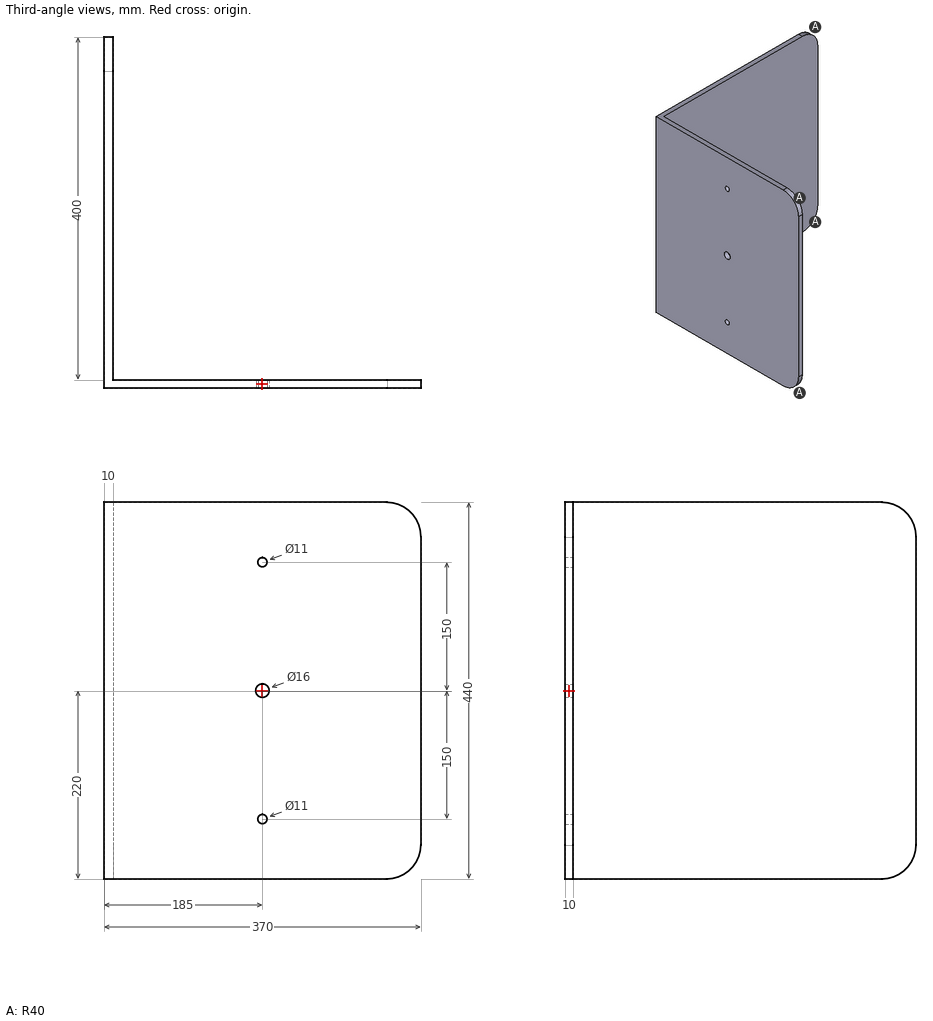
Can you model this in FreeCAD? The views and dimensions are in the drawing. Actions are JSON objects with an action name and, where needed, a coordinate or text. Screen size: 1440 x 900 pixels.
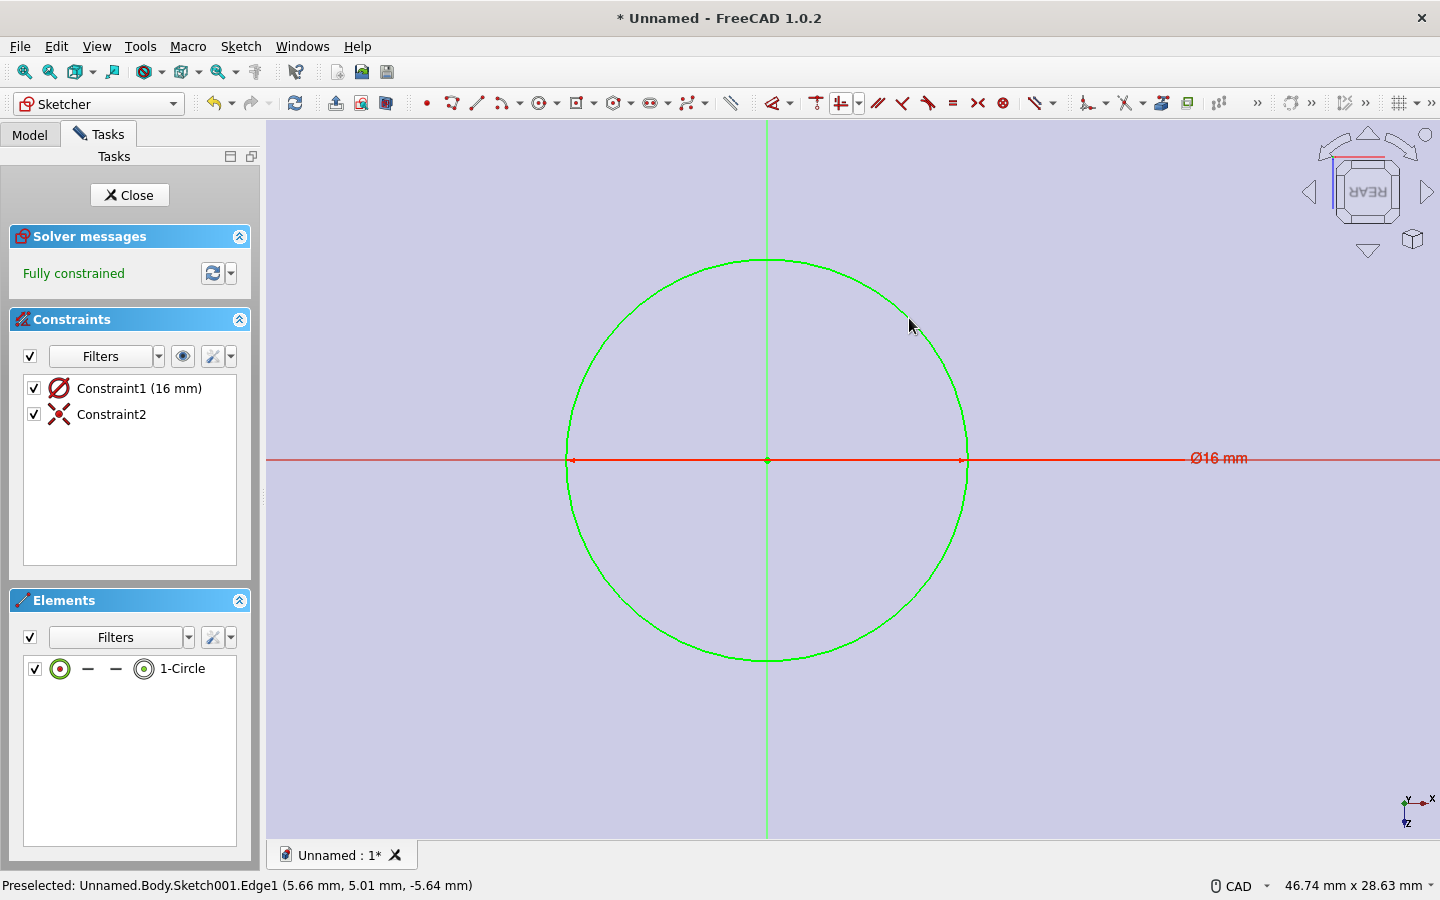
{"action": "left_click", "coordinate": [130, 195]}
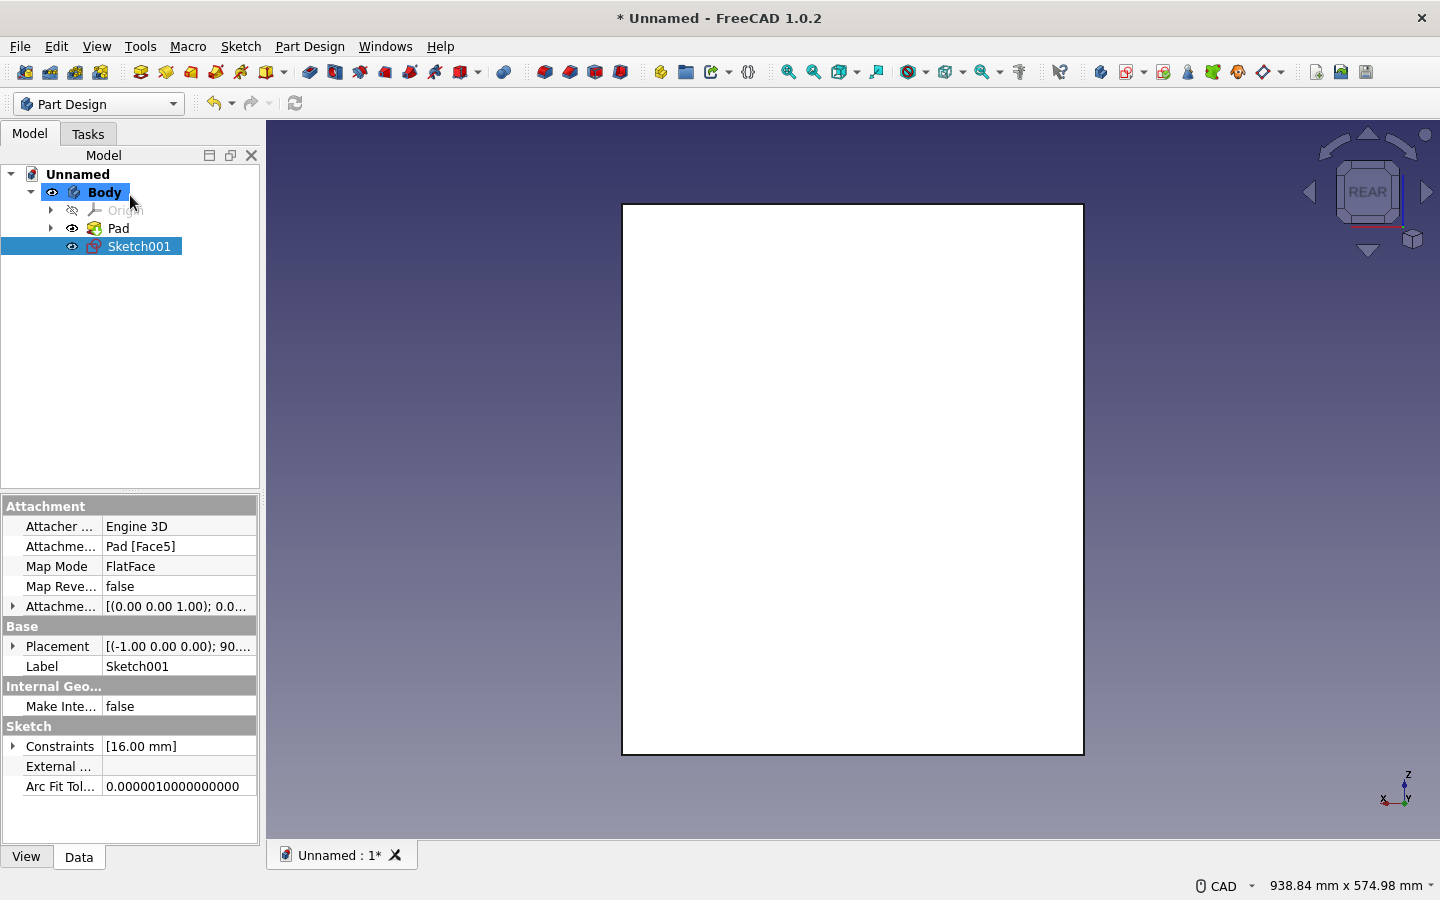
{"action": "left_click", "coordinate": [310, 72]}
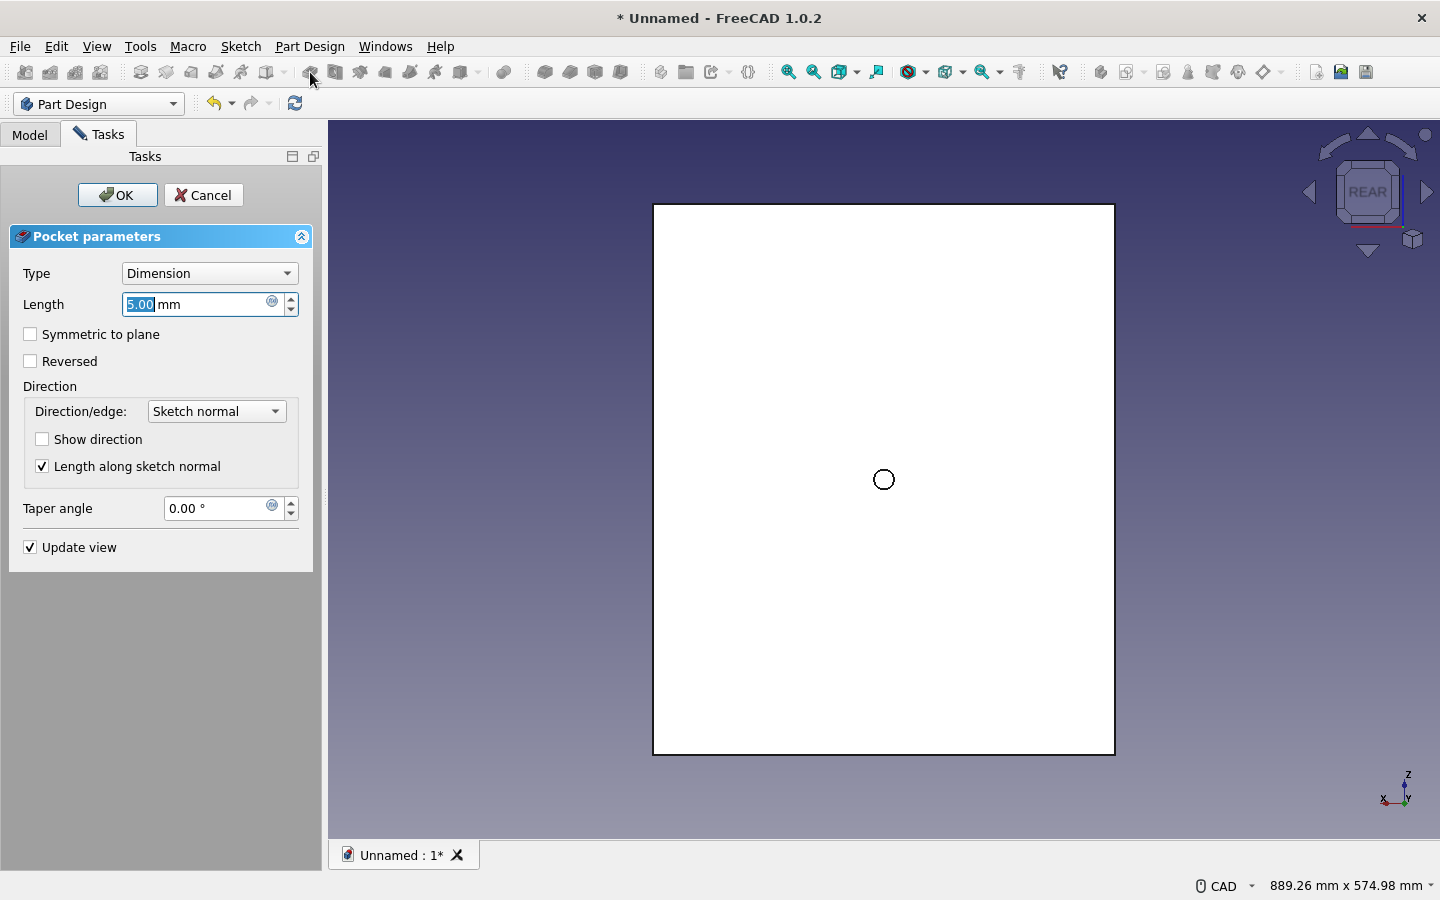
{"action": "left_click", "coordinate": [210, 274]}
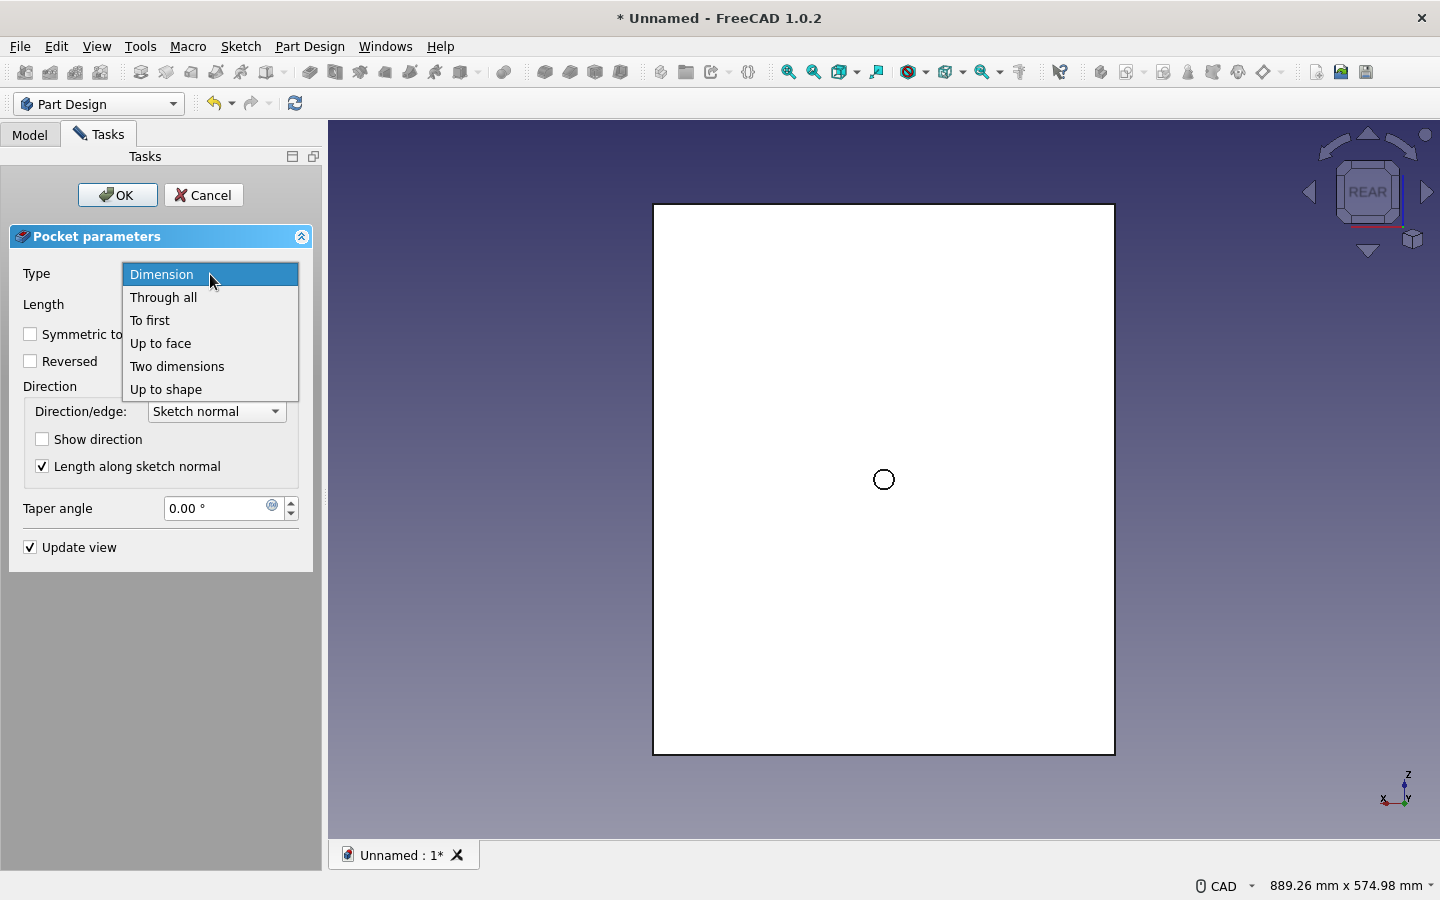
{"action": "left_click", "coordinate": [208, 320]}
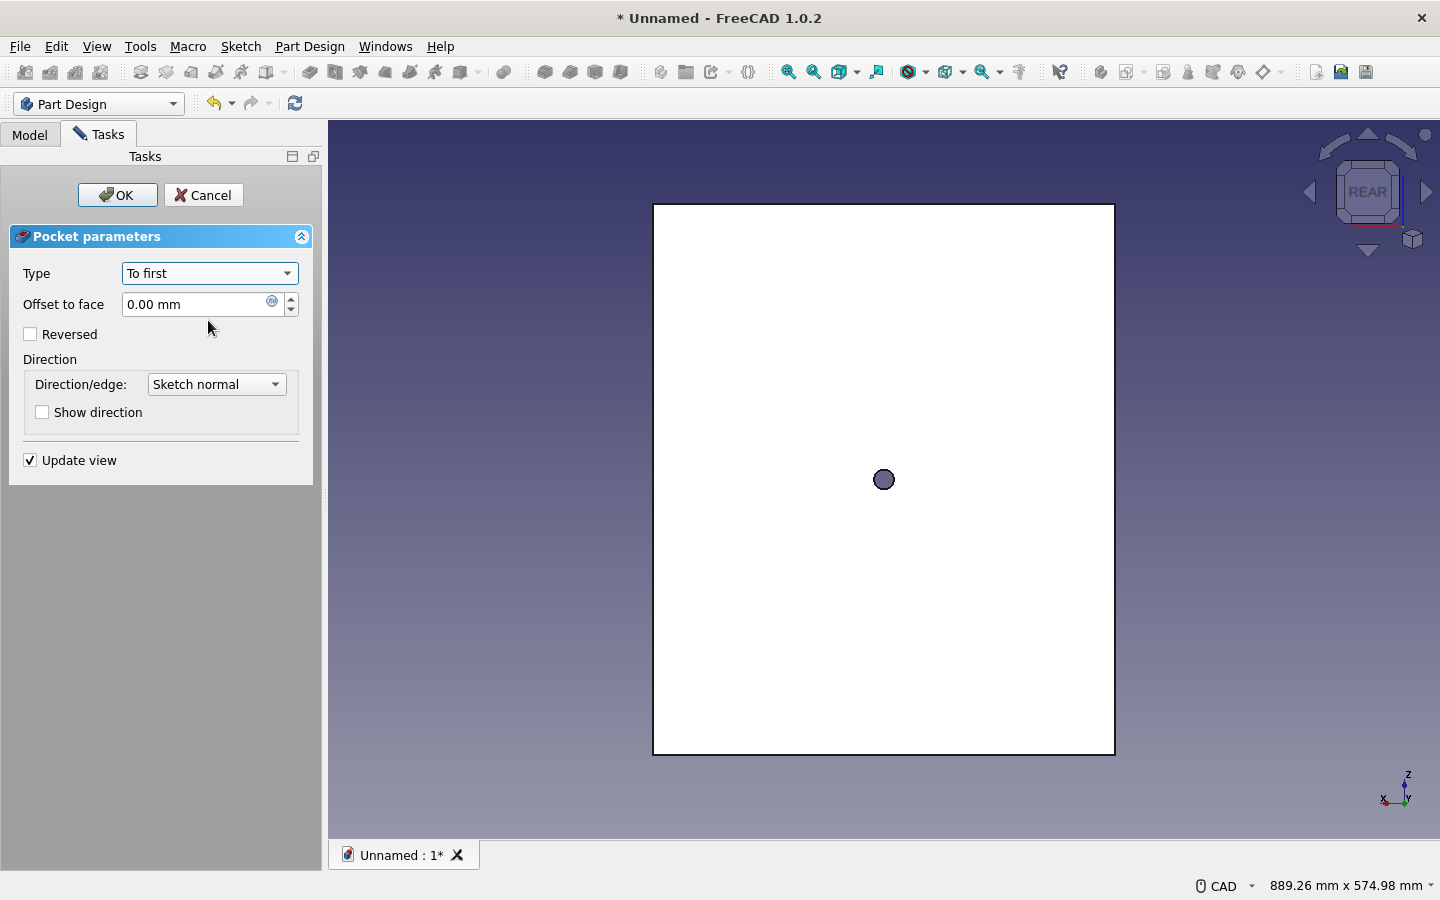
{"action": "left_click", "coordinate": [118, 195]}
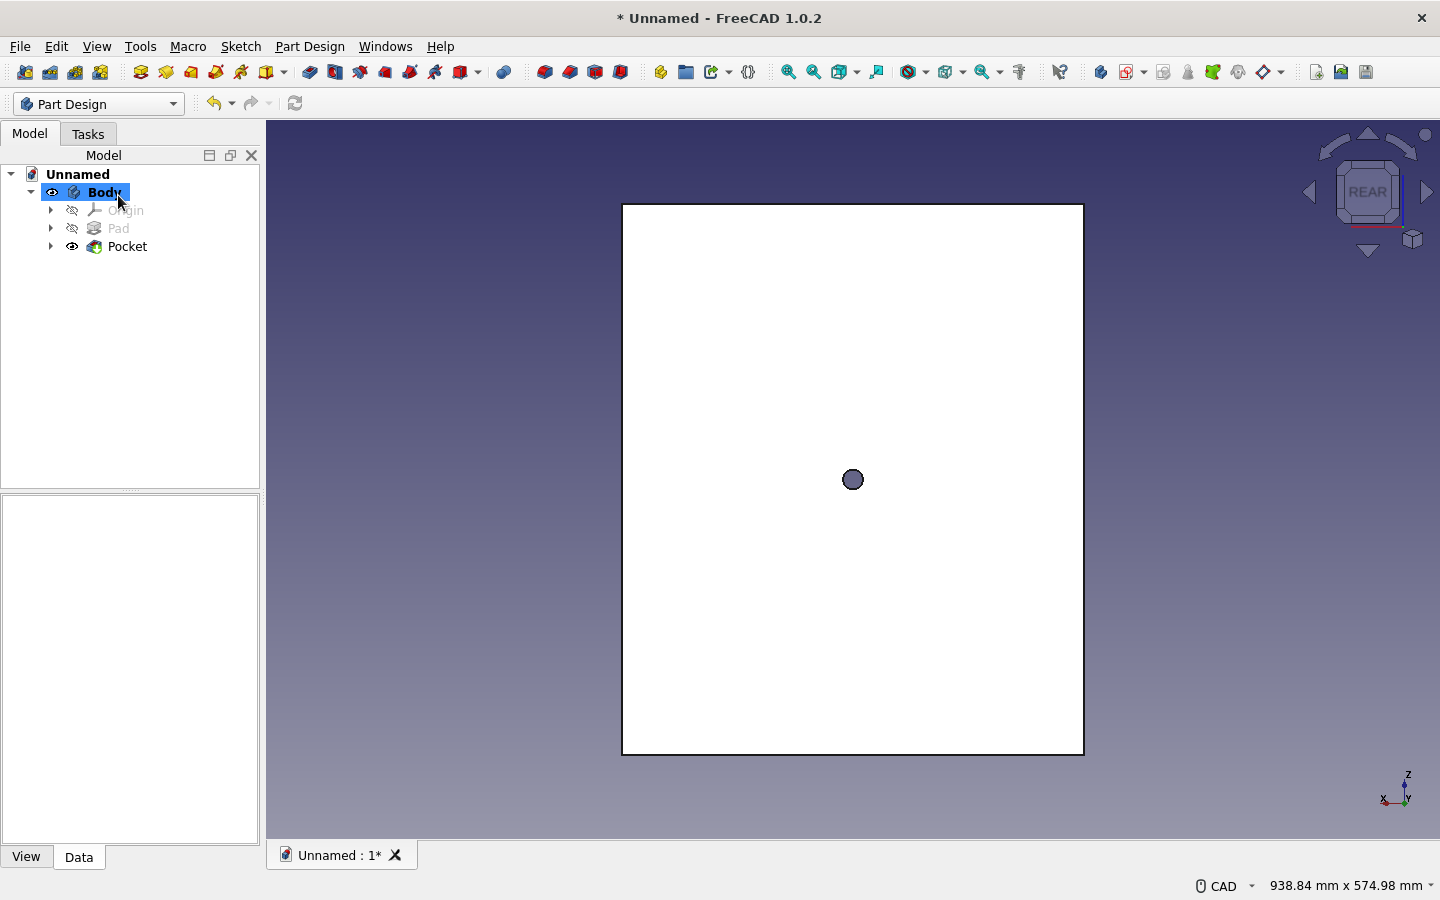
{"action": "left_click", "coordinate": [787, 636]}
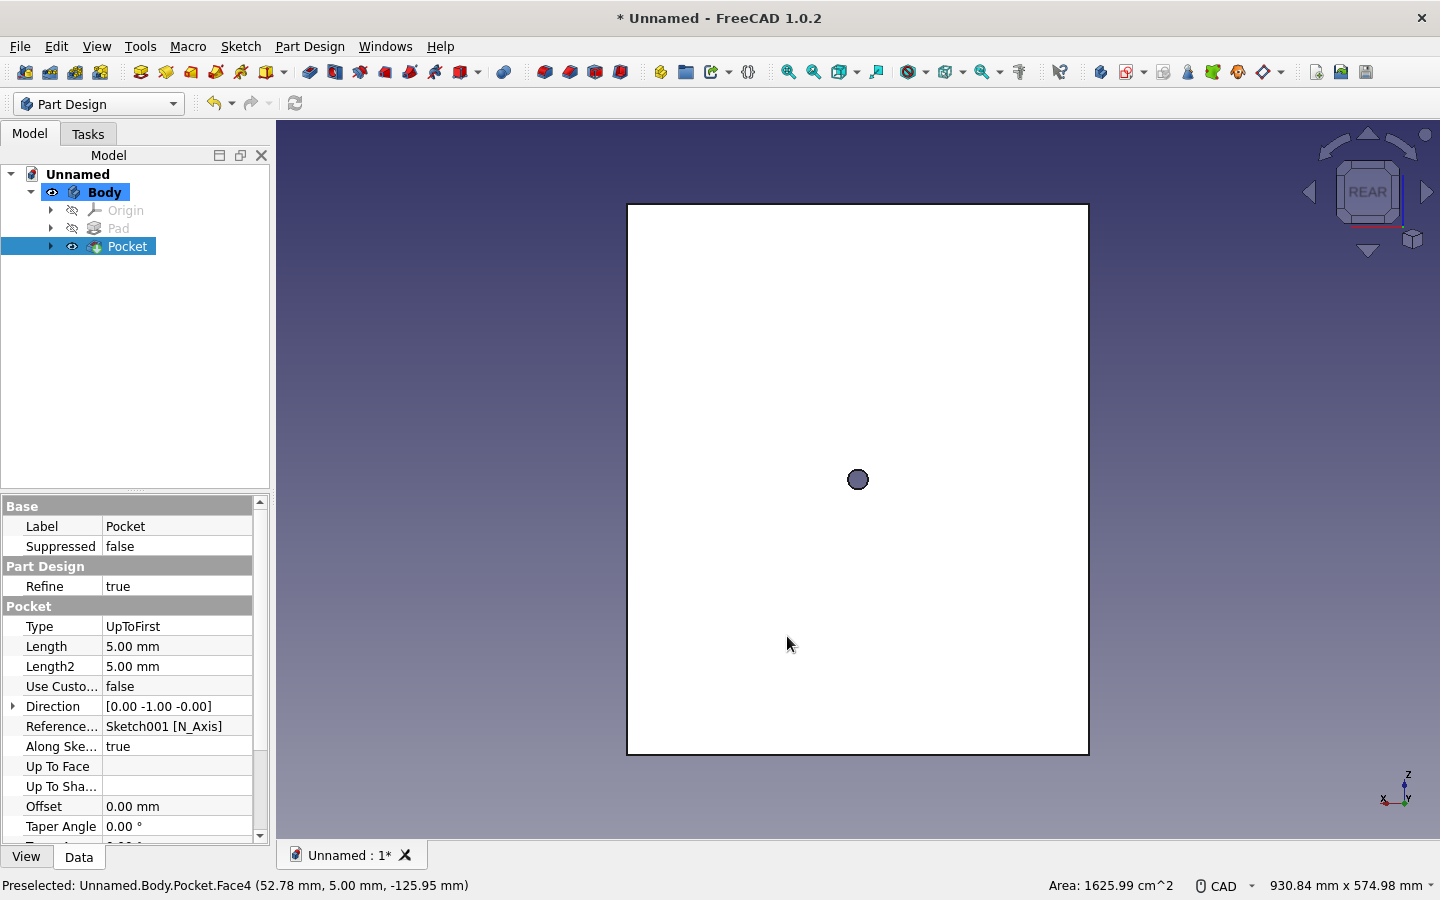
{"action": "left_click", "coordinate": [1126, 72]}